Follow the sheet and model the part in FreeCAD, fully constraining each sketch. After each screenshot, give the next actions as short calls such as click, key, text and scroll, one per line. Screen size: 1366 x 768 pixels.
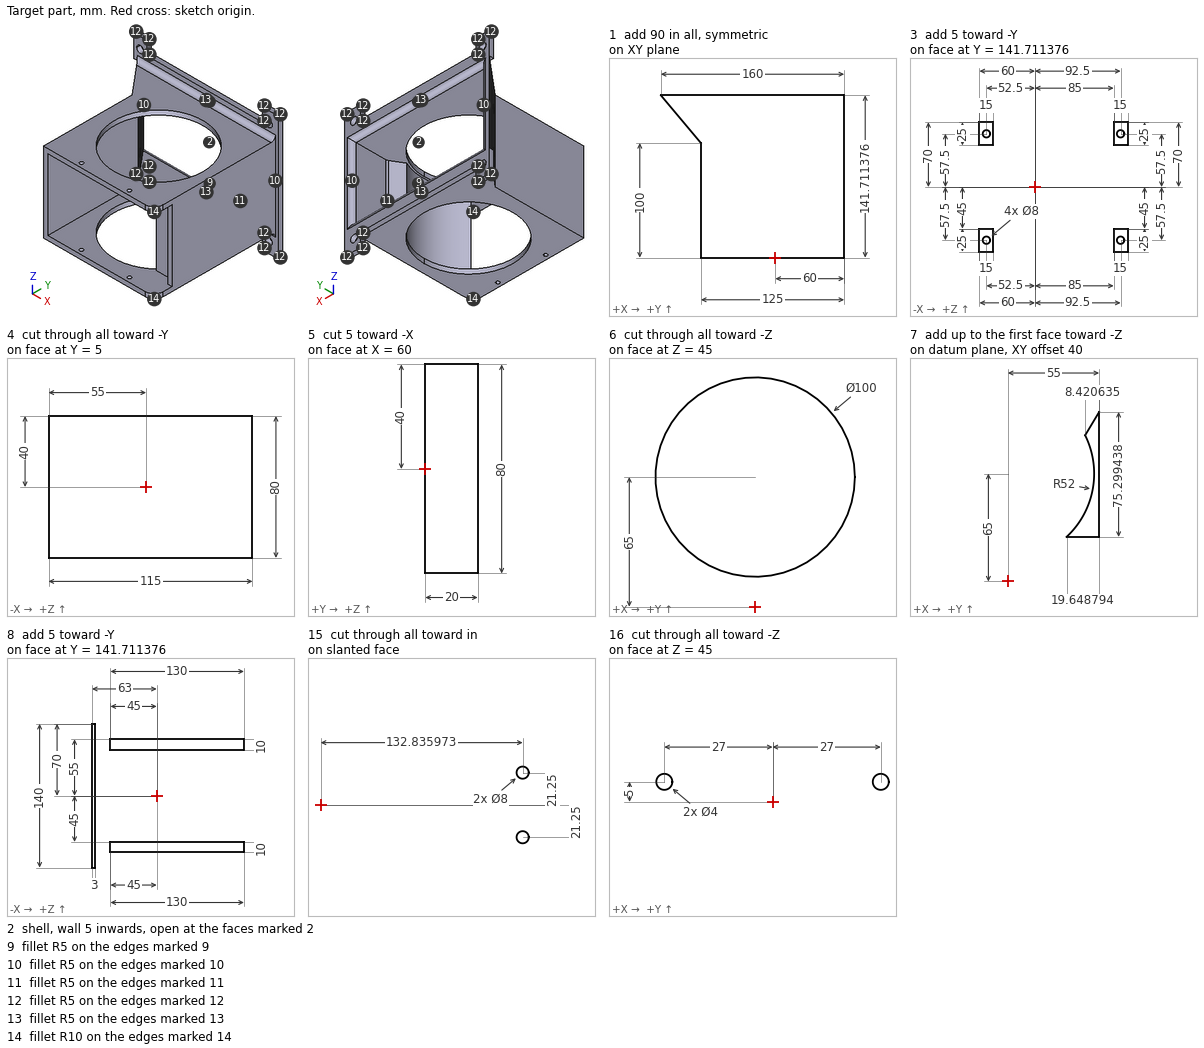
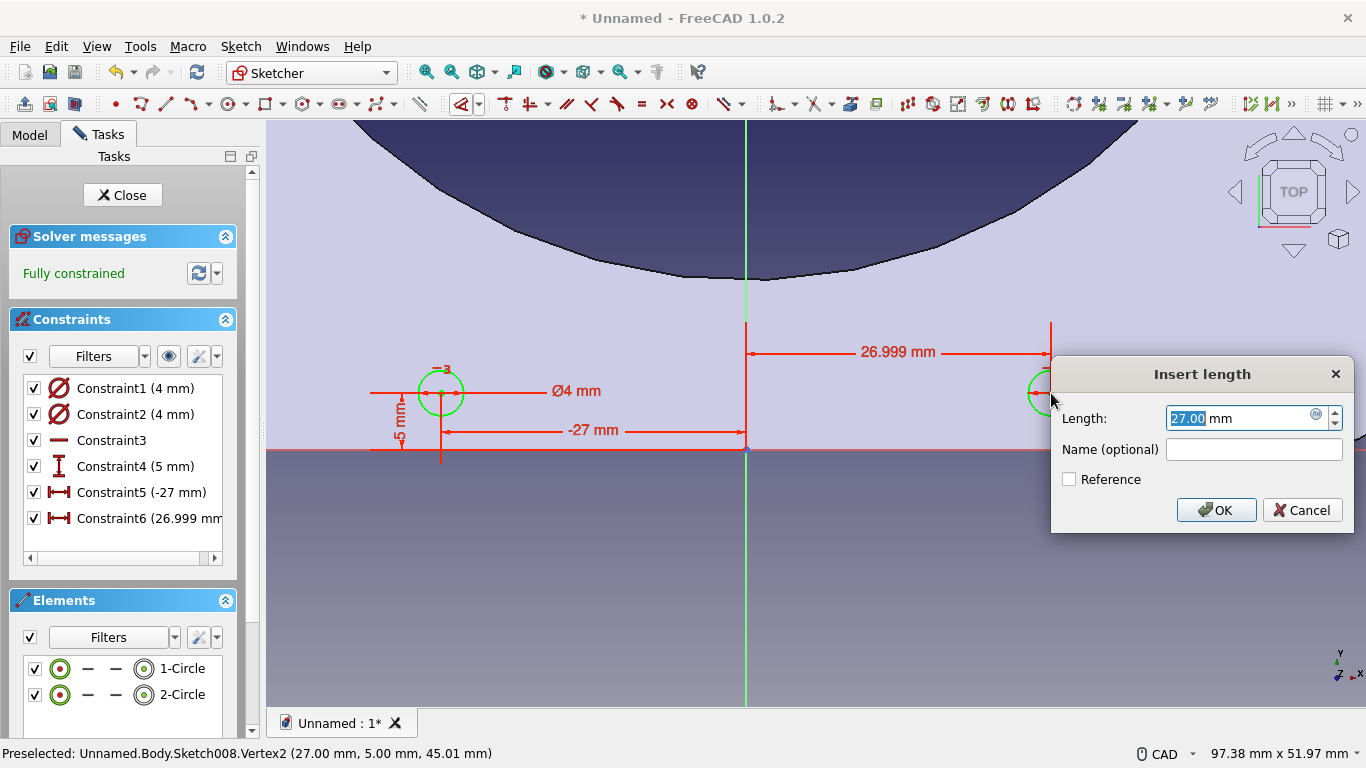
text(27)
key(Return)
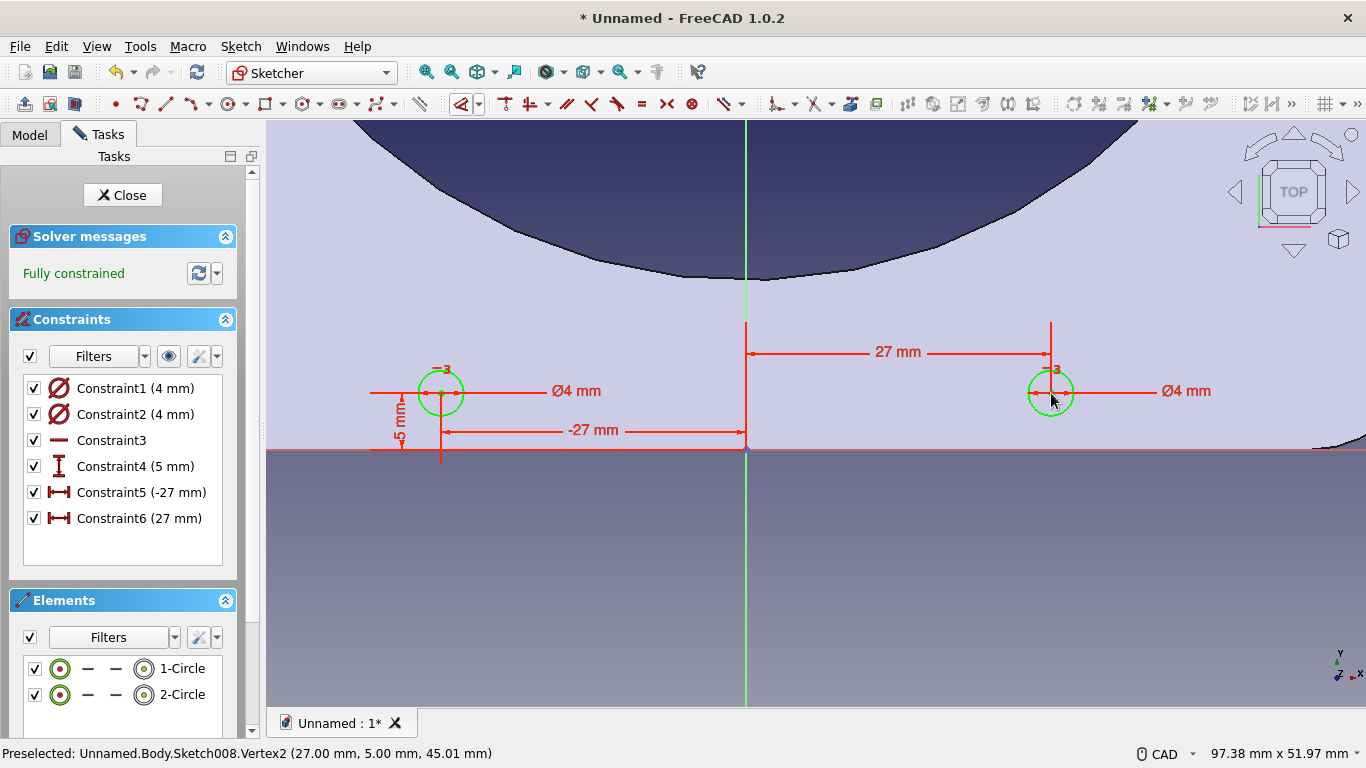
click(123, 195)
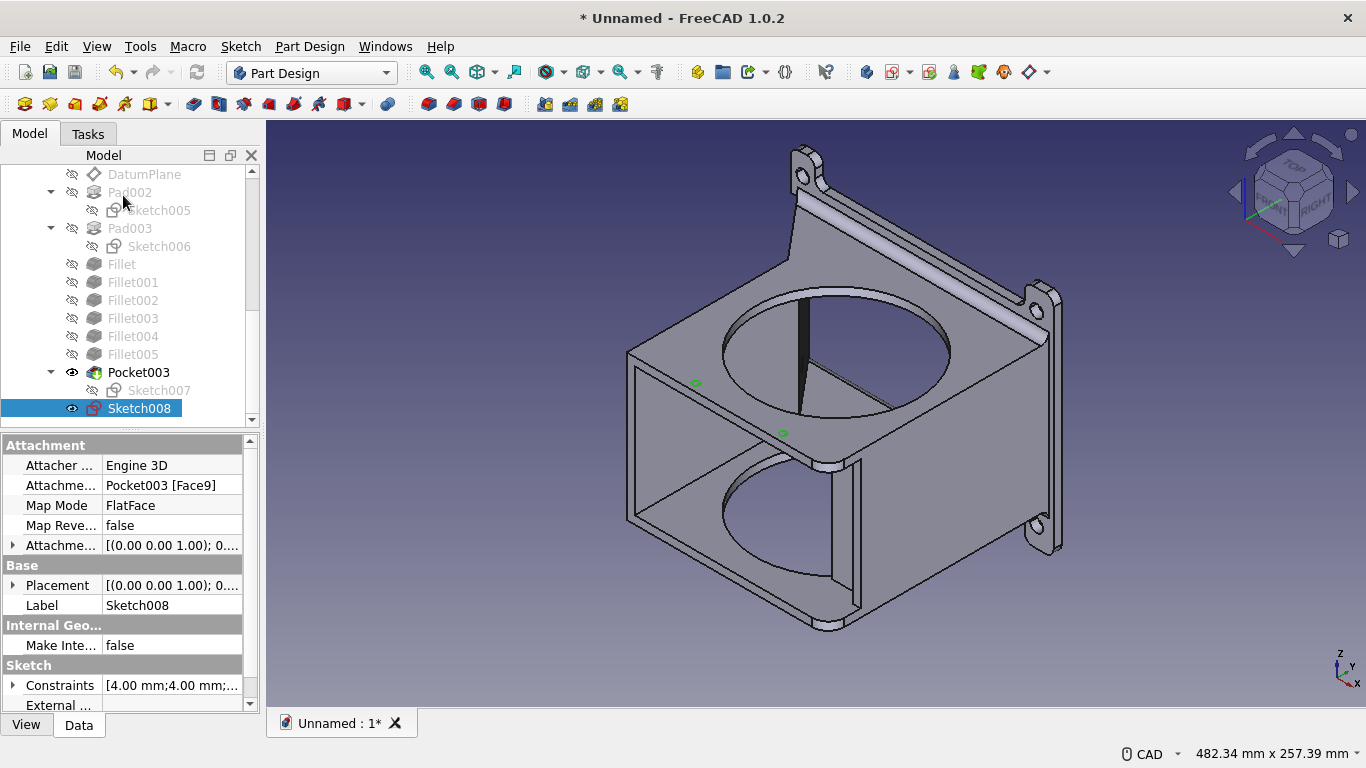
click(194, 104)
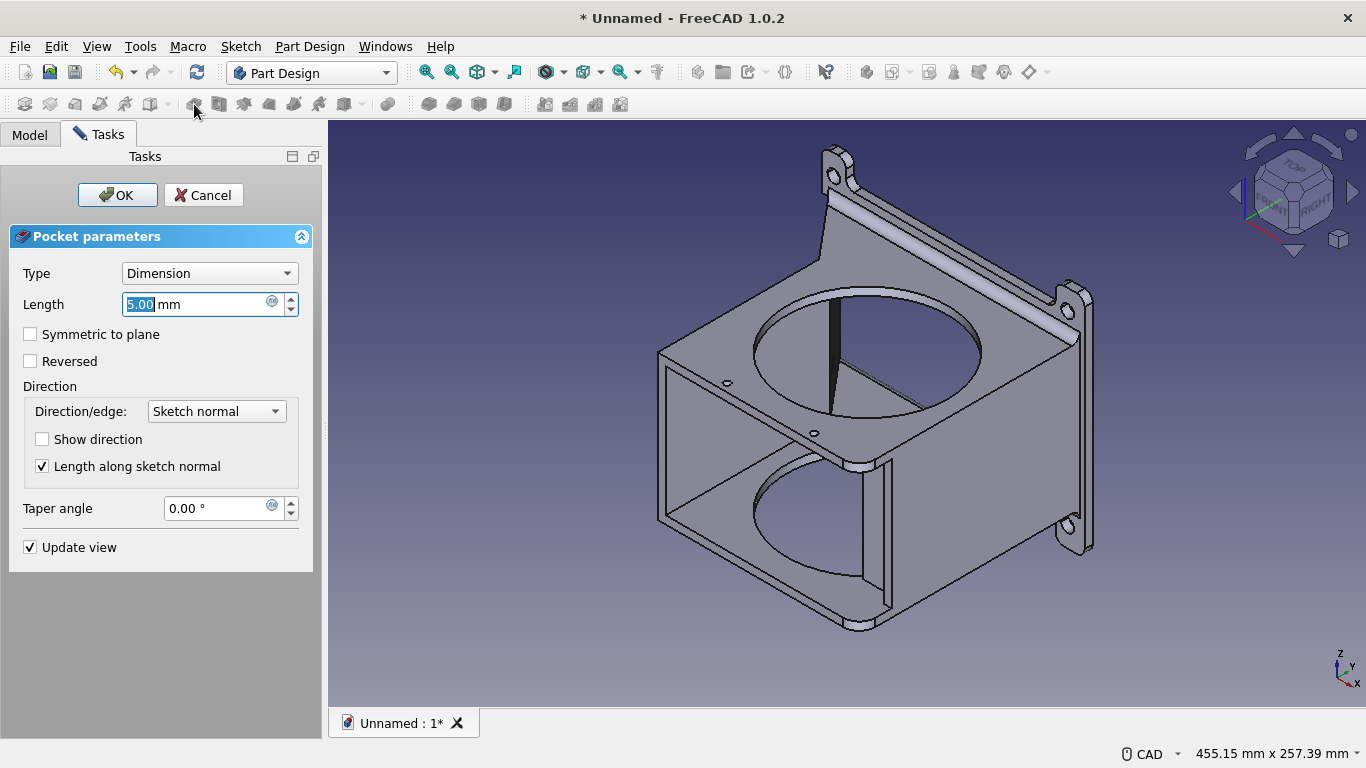
click(210, 274)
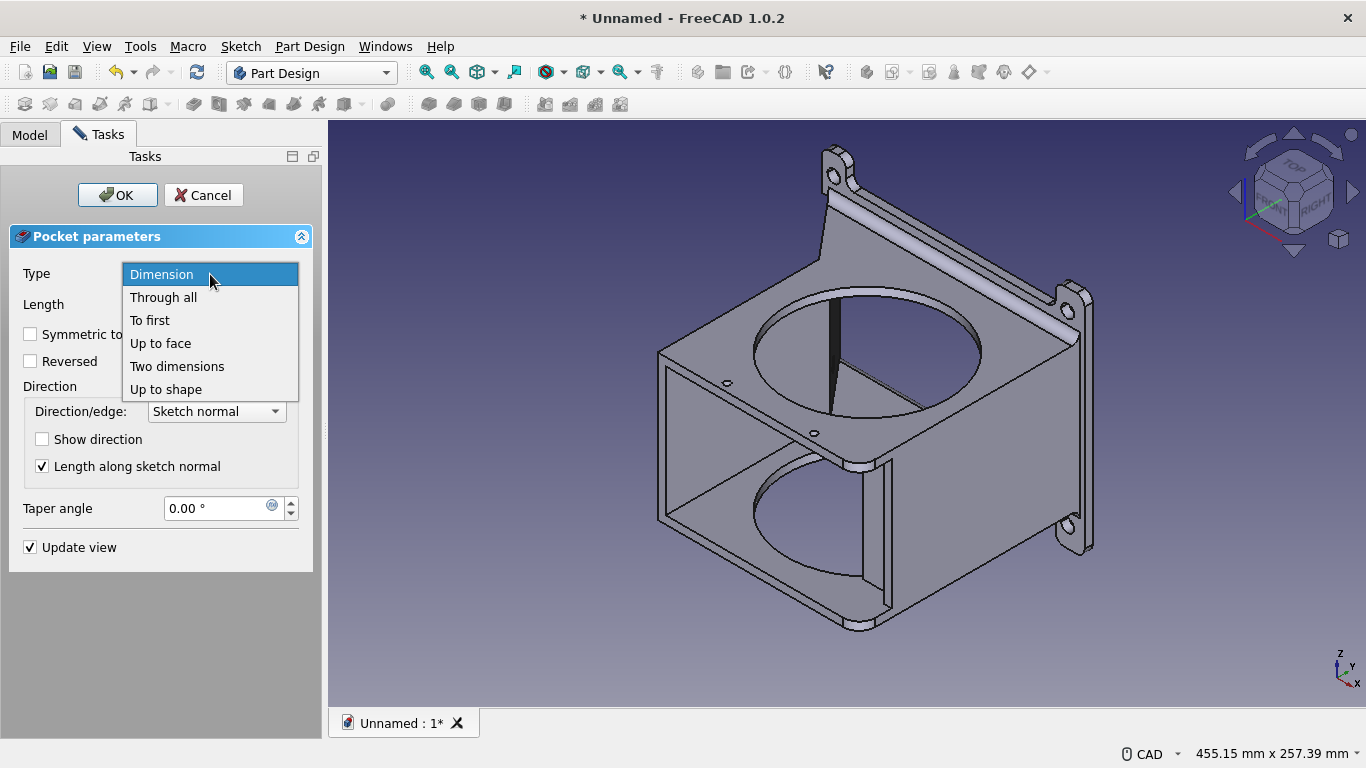
click(208, 298)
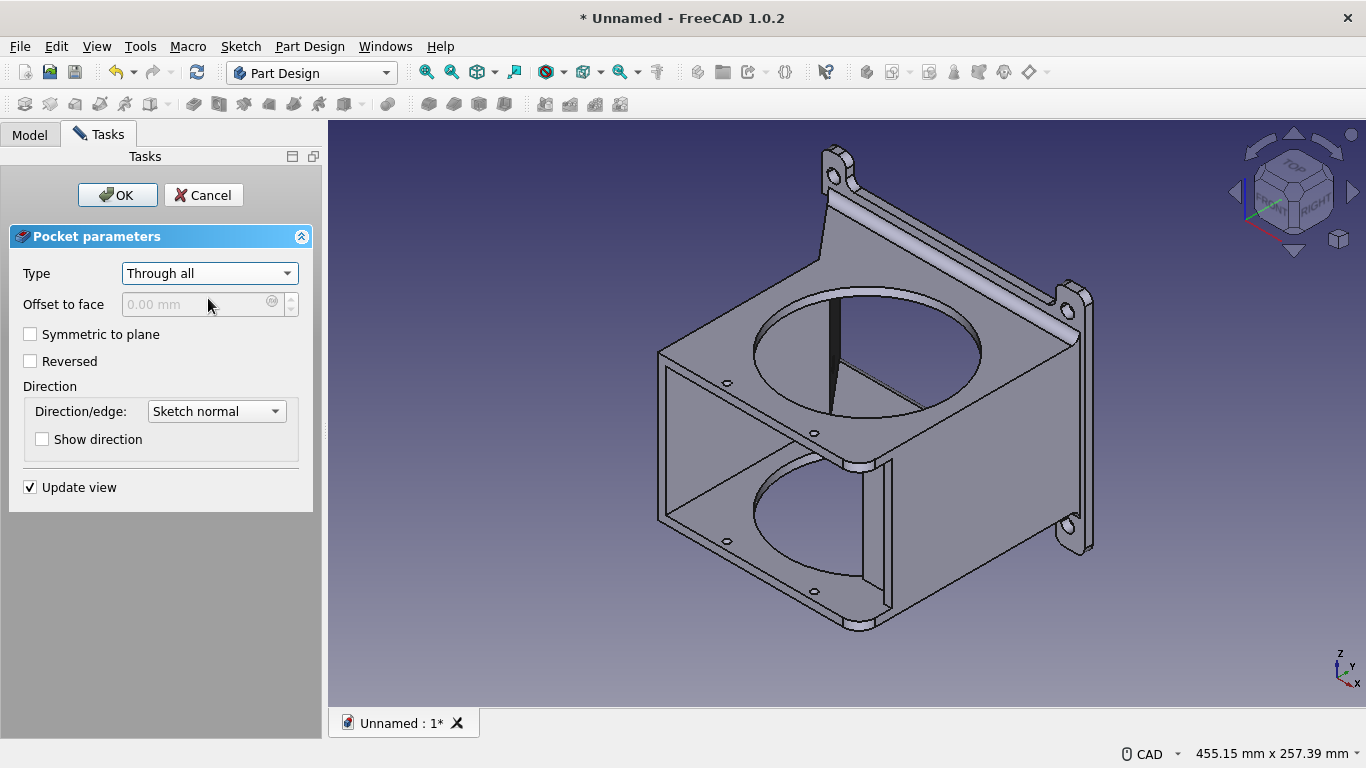
click(118, 195)